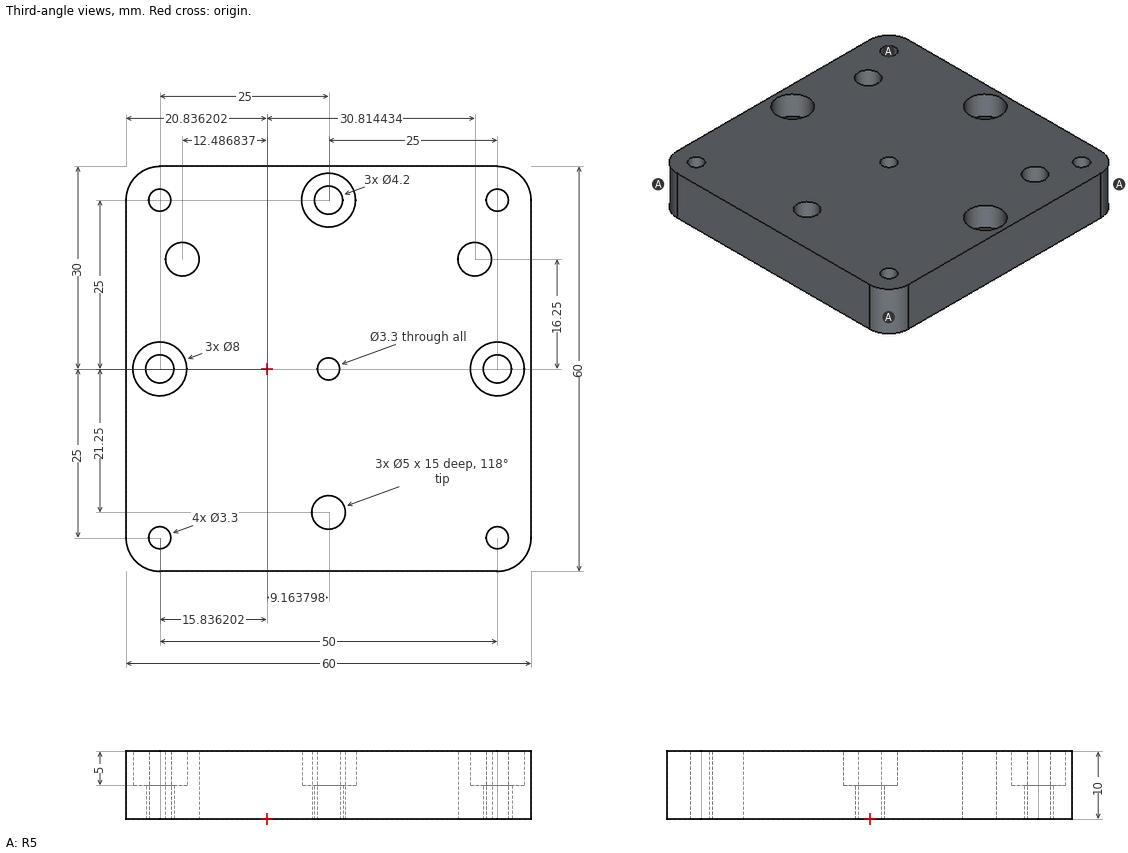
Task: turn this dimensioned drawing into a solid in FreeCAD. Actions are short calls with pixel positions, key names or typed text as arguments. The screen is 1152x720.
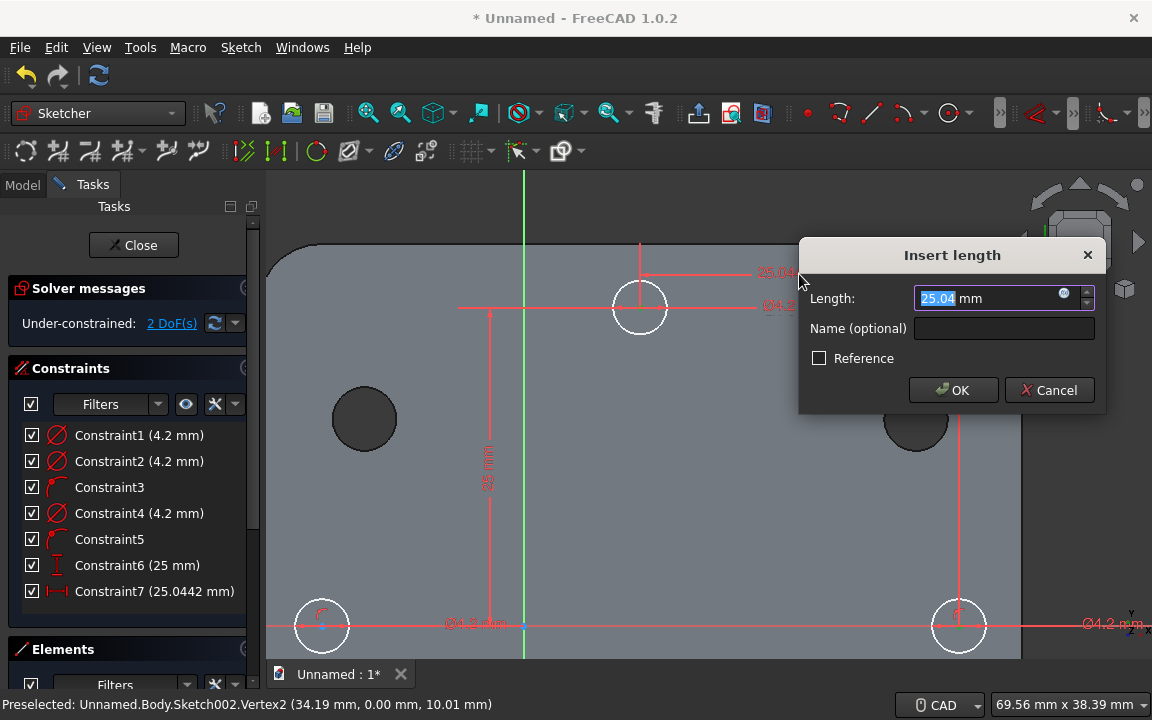
text(25)
key(Return)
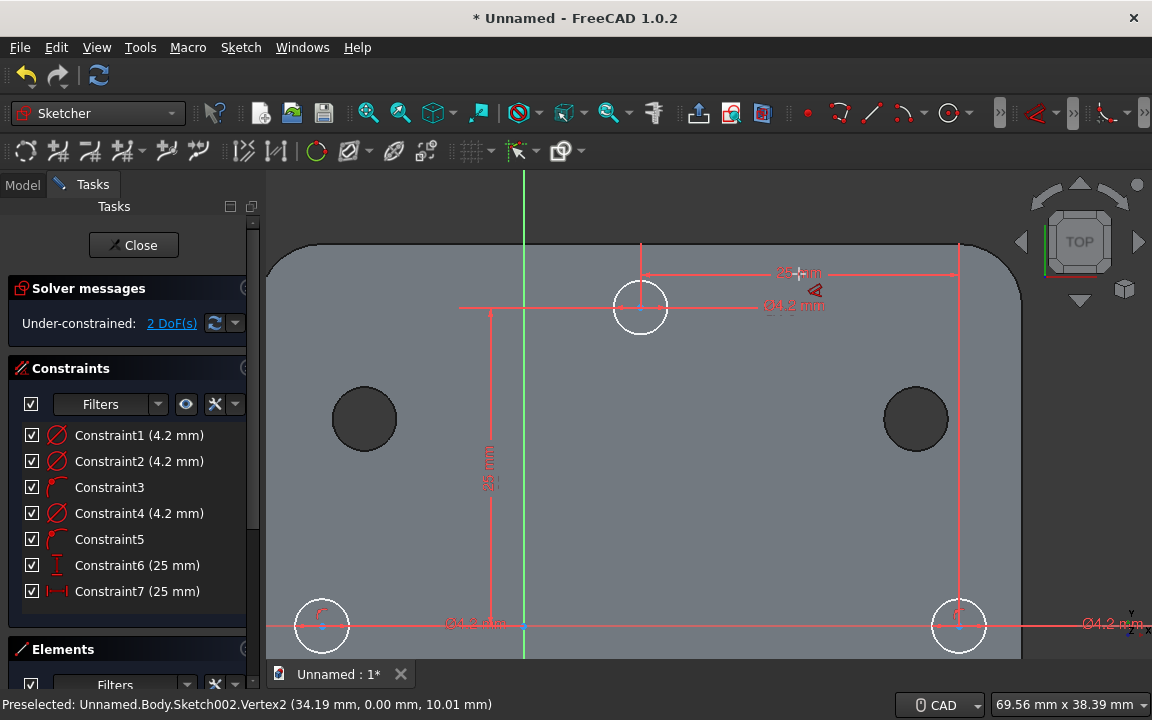
click(641, 308)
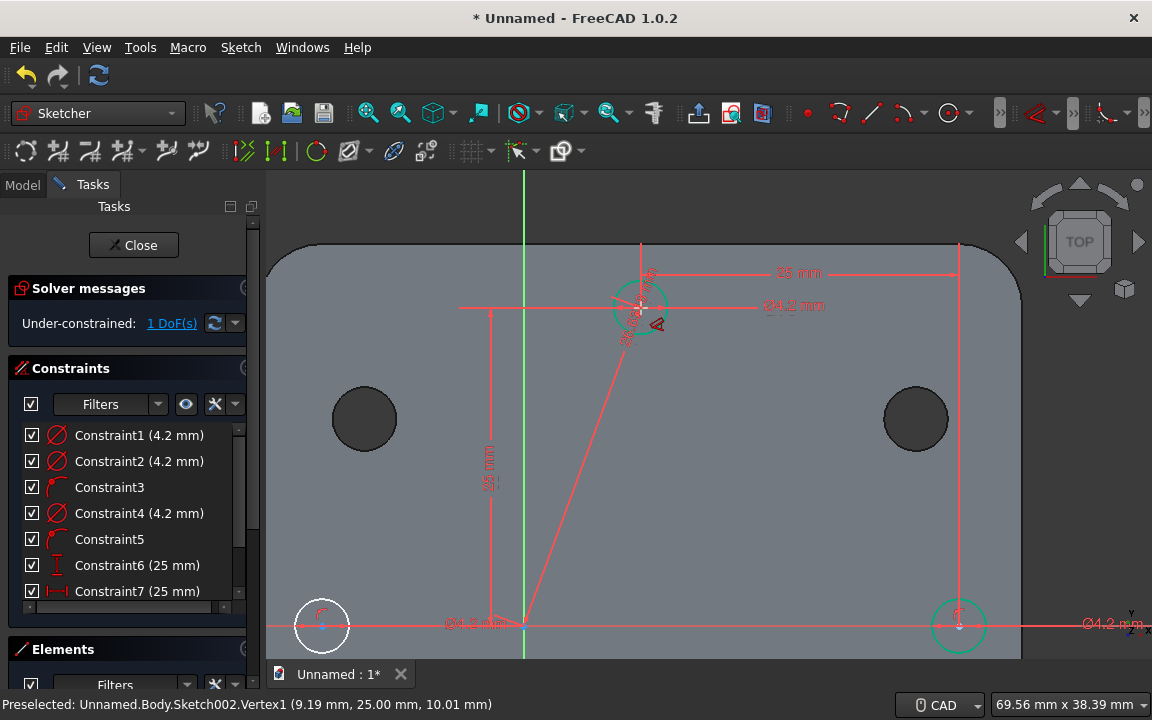
click(322, 626)
click(481, 274)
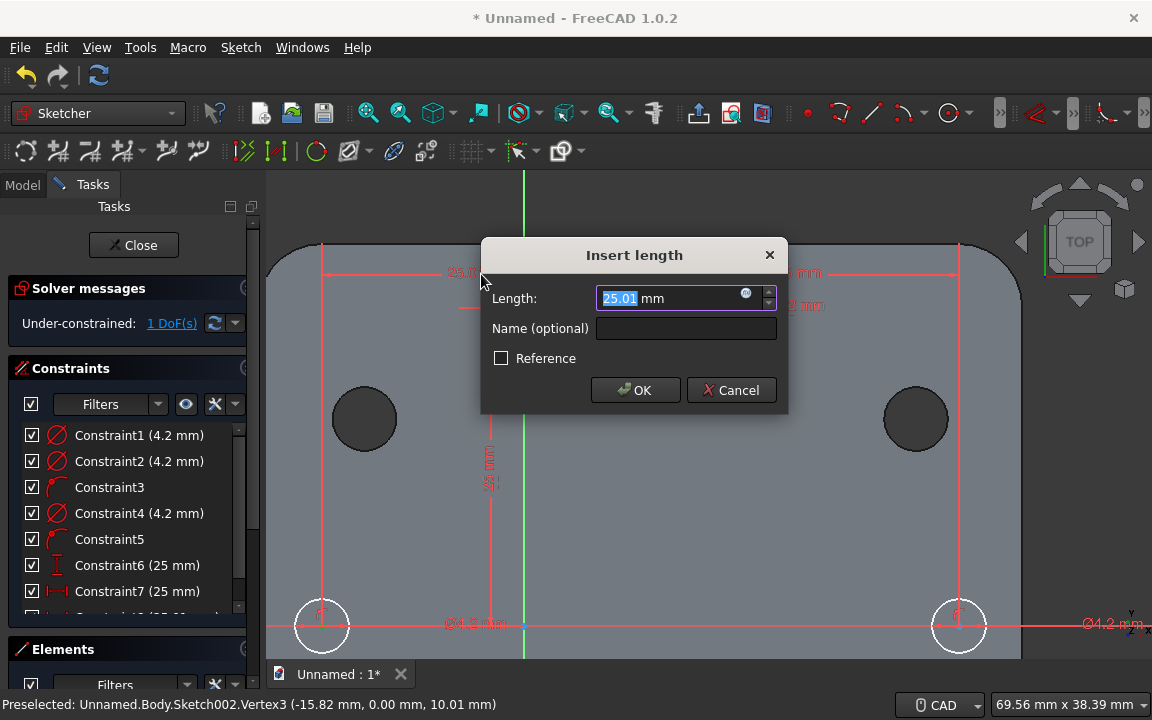
text(25)
key(Return)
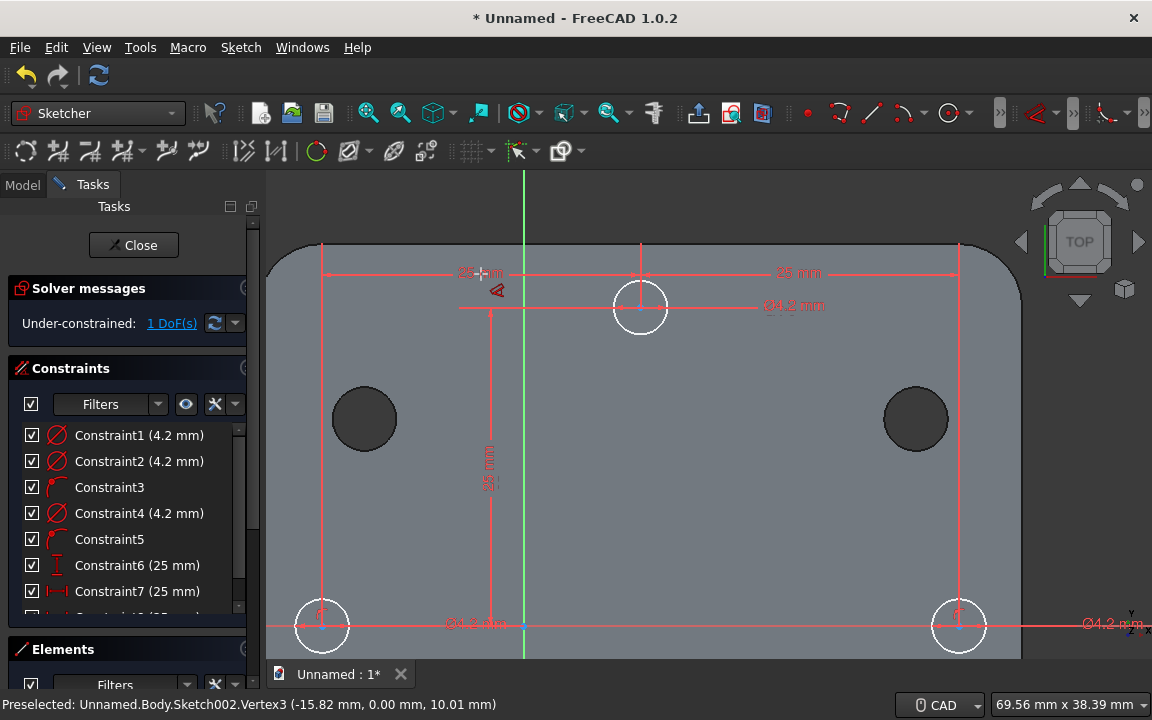
click(641, 308)
click(582, 274)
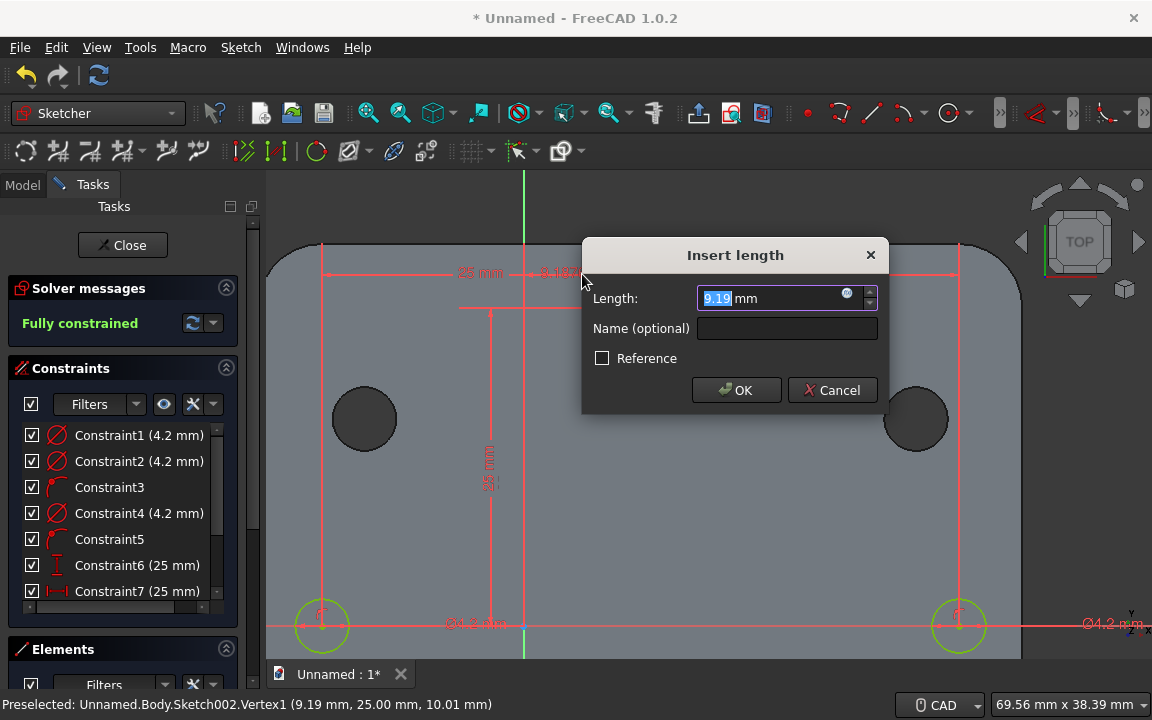
text(9.163798)
key(Return)
key(Escape)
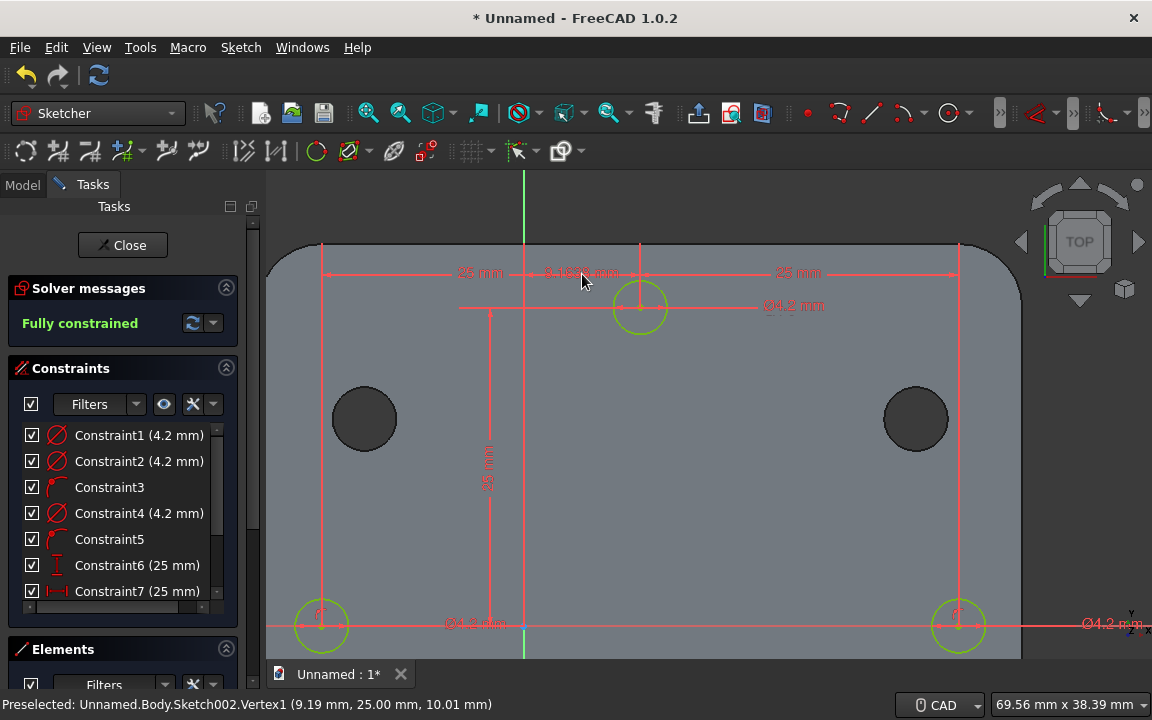
click(123, 245)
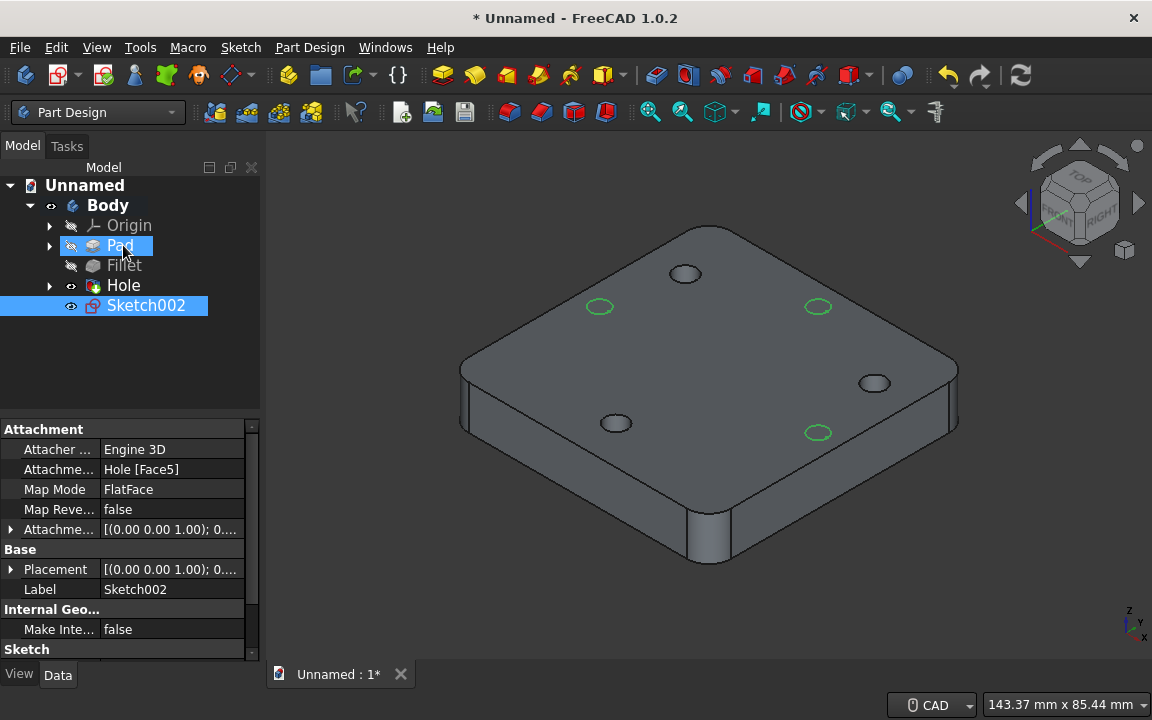
click(658, 76)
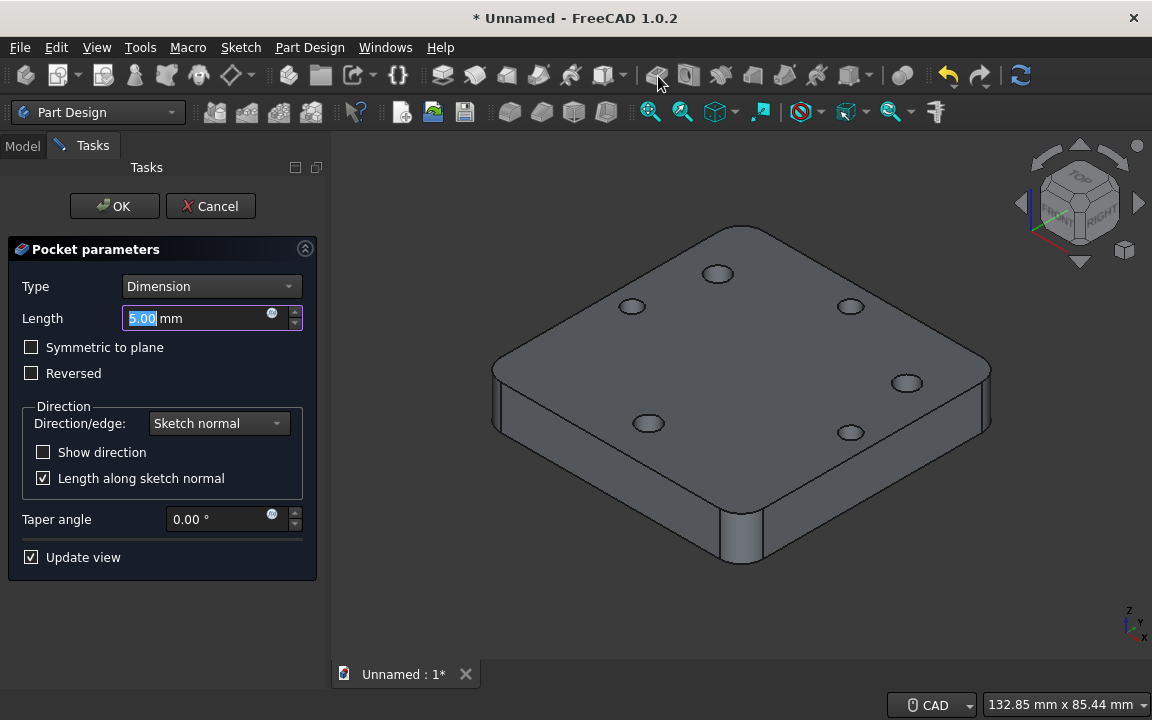
click(212, 286)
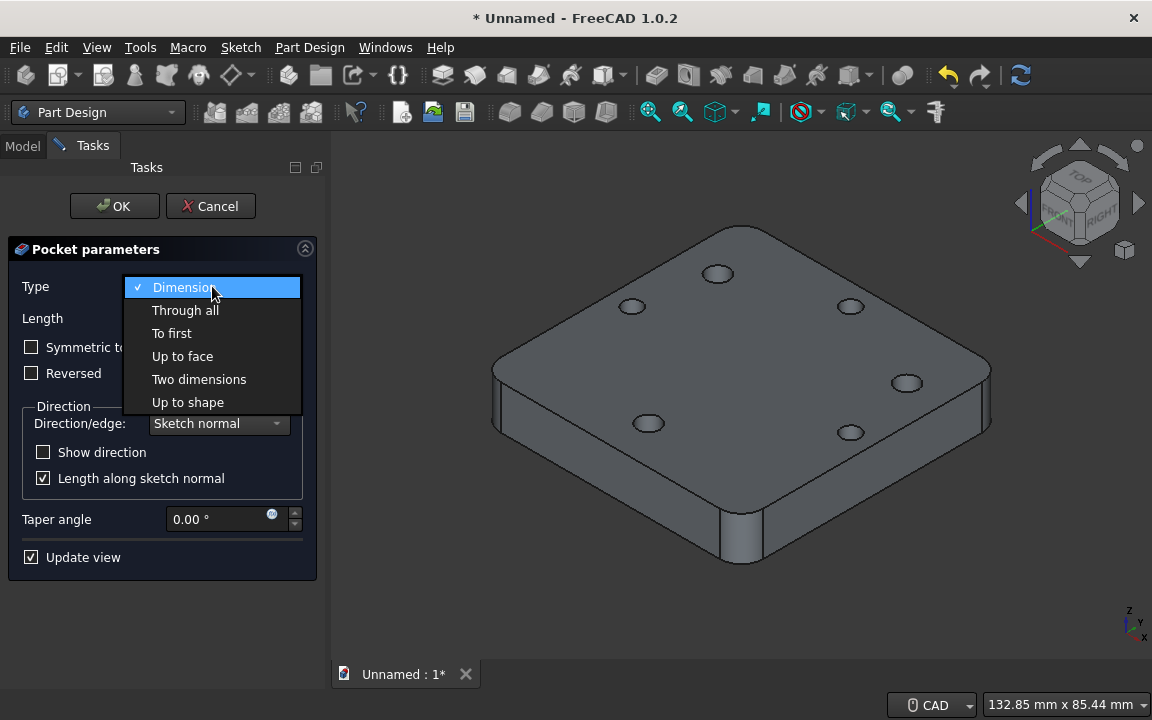
click(212, 310)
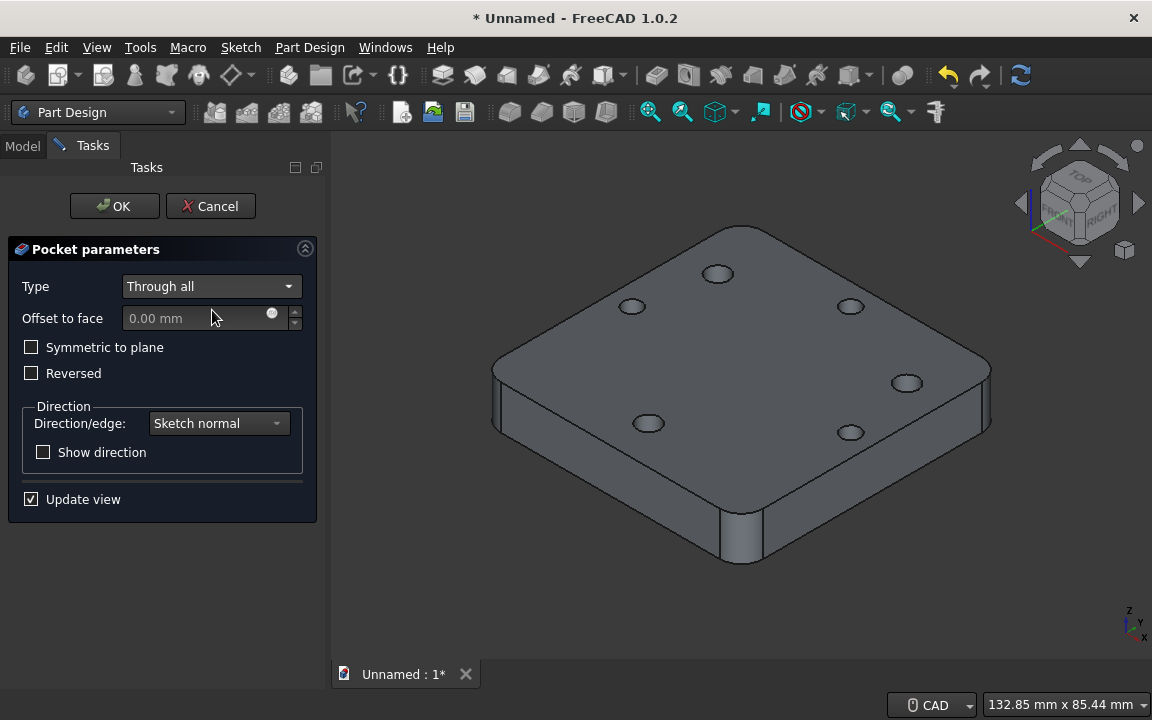
click(115, 206)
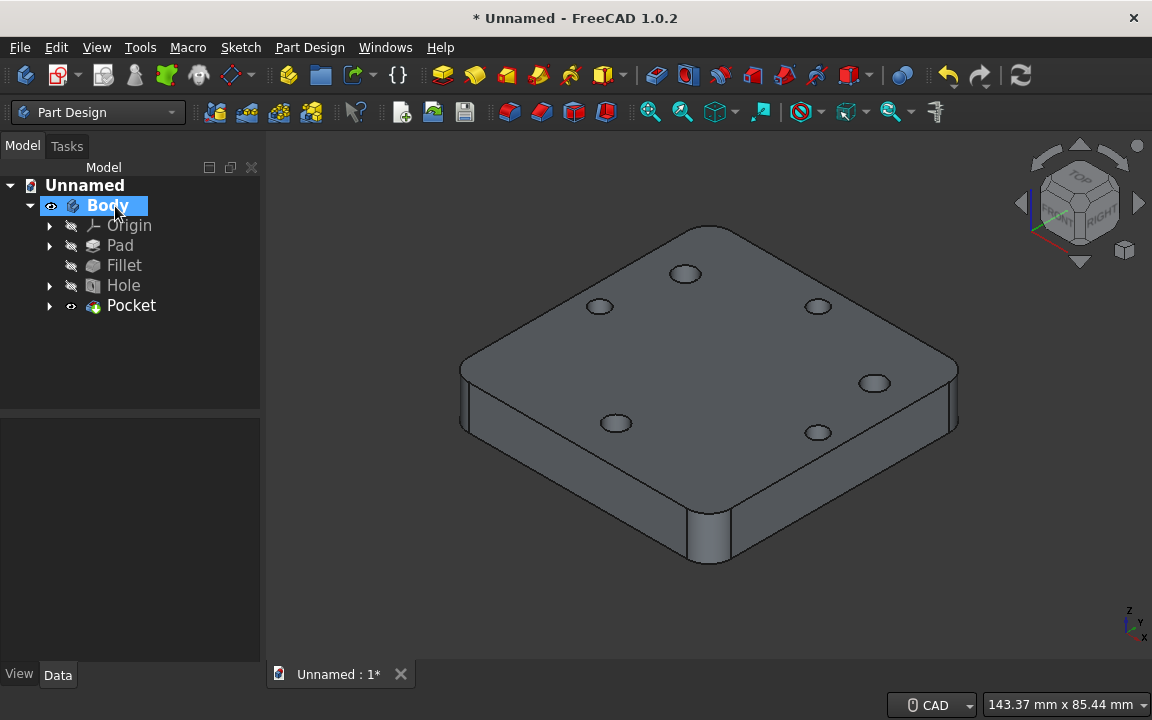
click(709, 369)